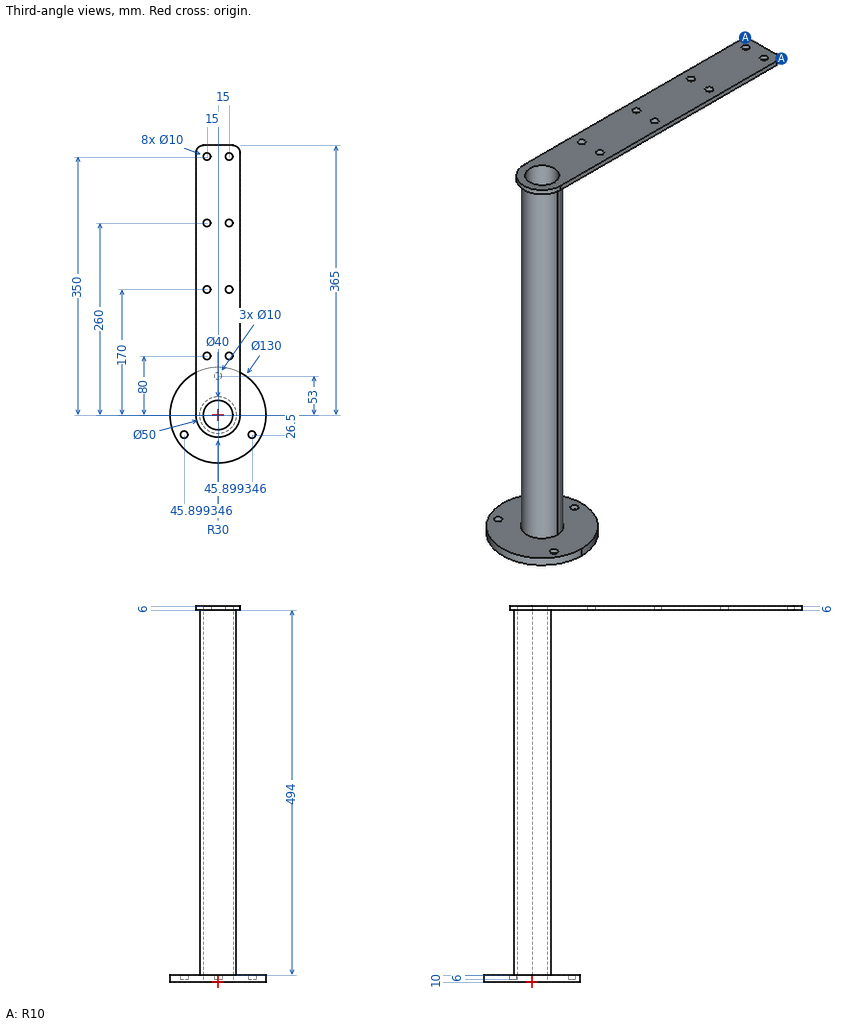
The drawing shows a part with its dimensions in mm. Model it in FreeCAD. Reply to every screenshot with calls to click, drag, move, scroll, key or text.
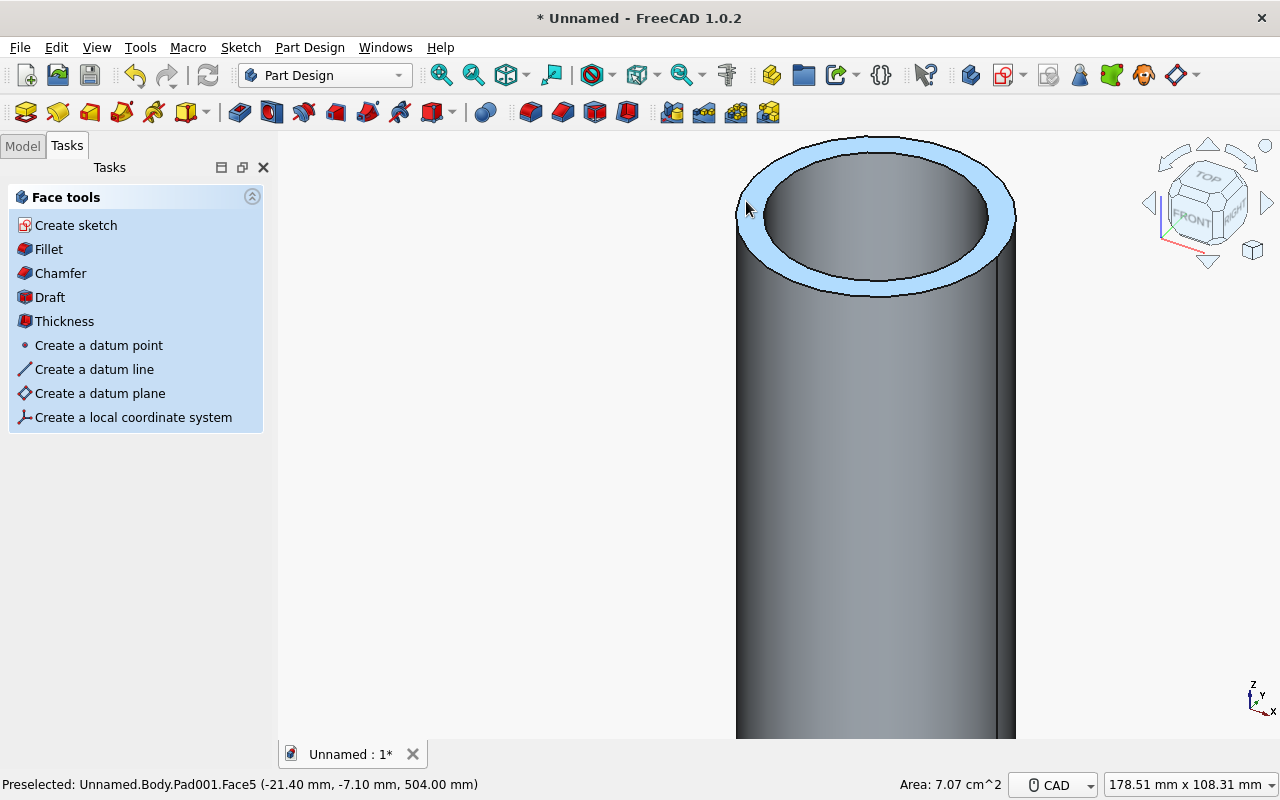
click(1004, 76)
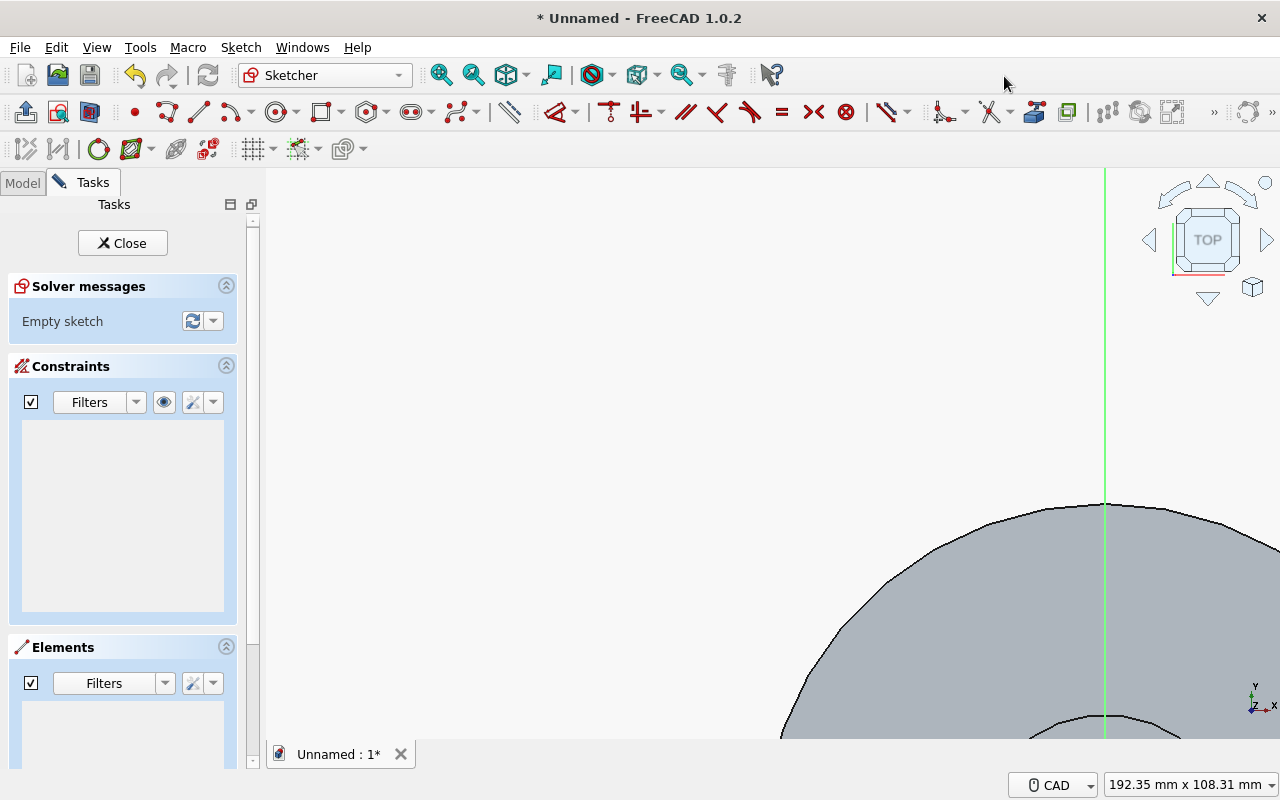
scroll(625, 551, down, 9)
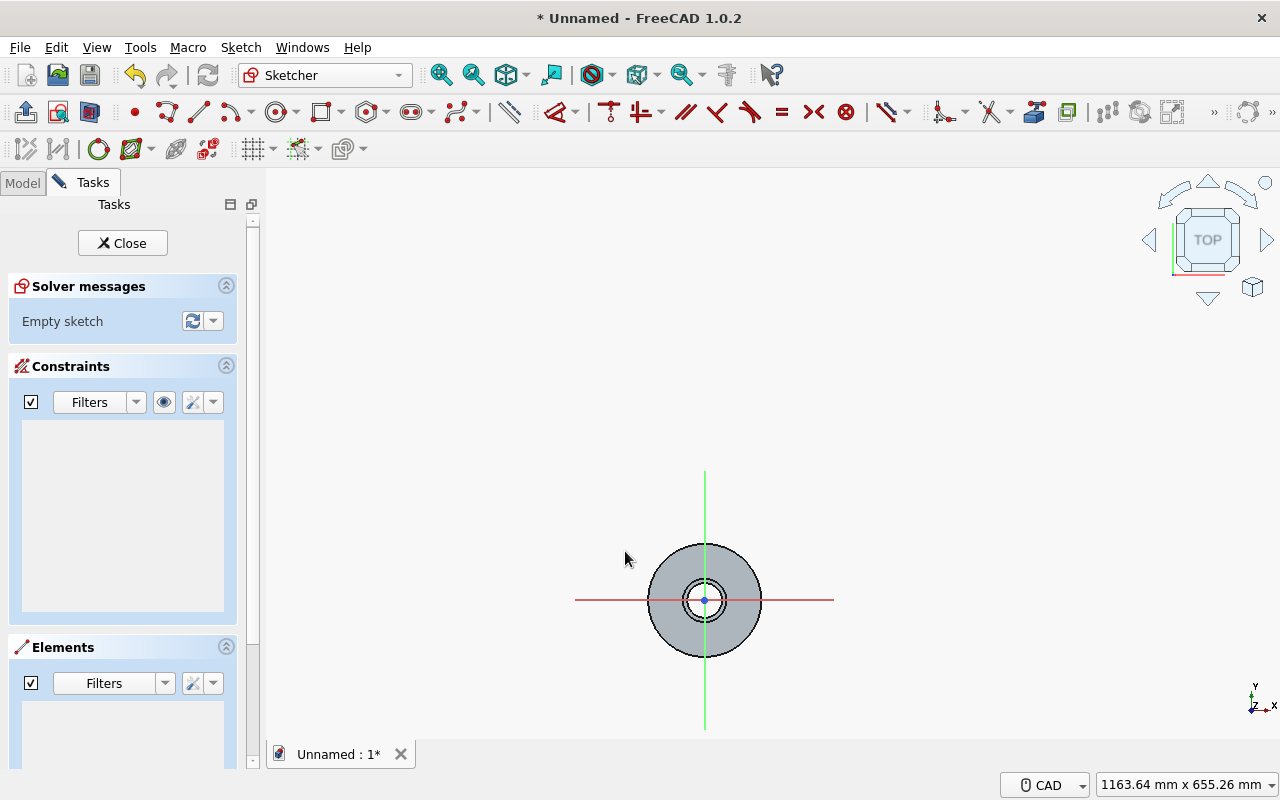
click(168, 112)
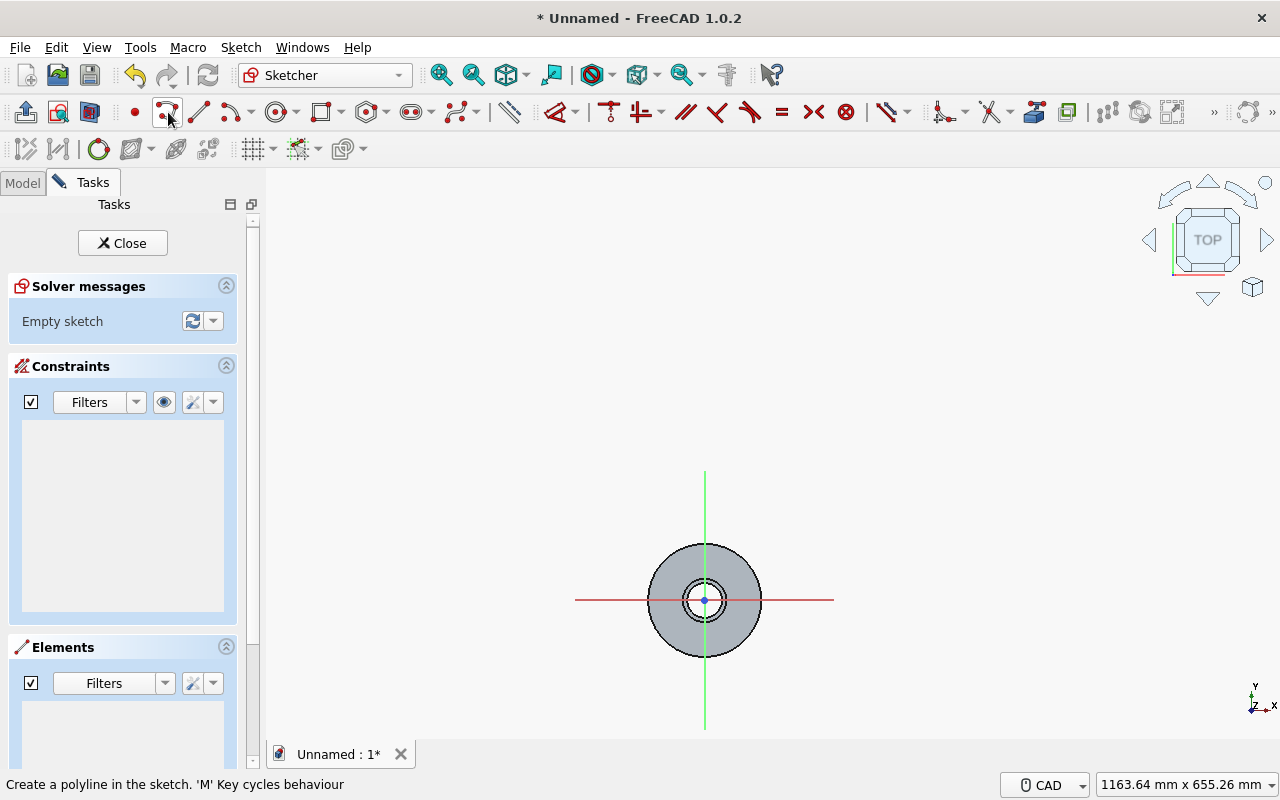
click(731, 600)
click(731, 282)
click(679, 282)
click(679, 600)
right_click(679, 600)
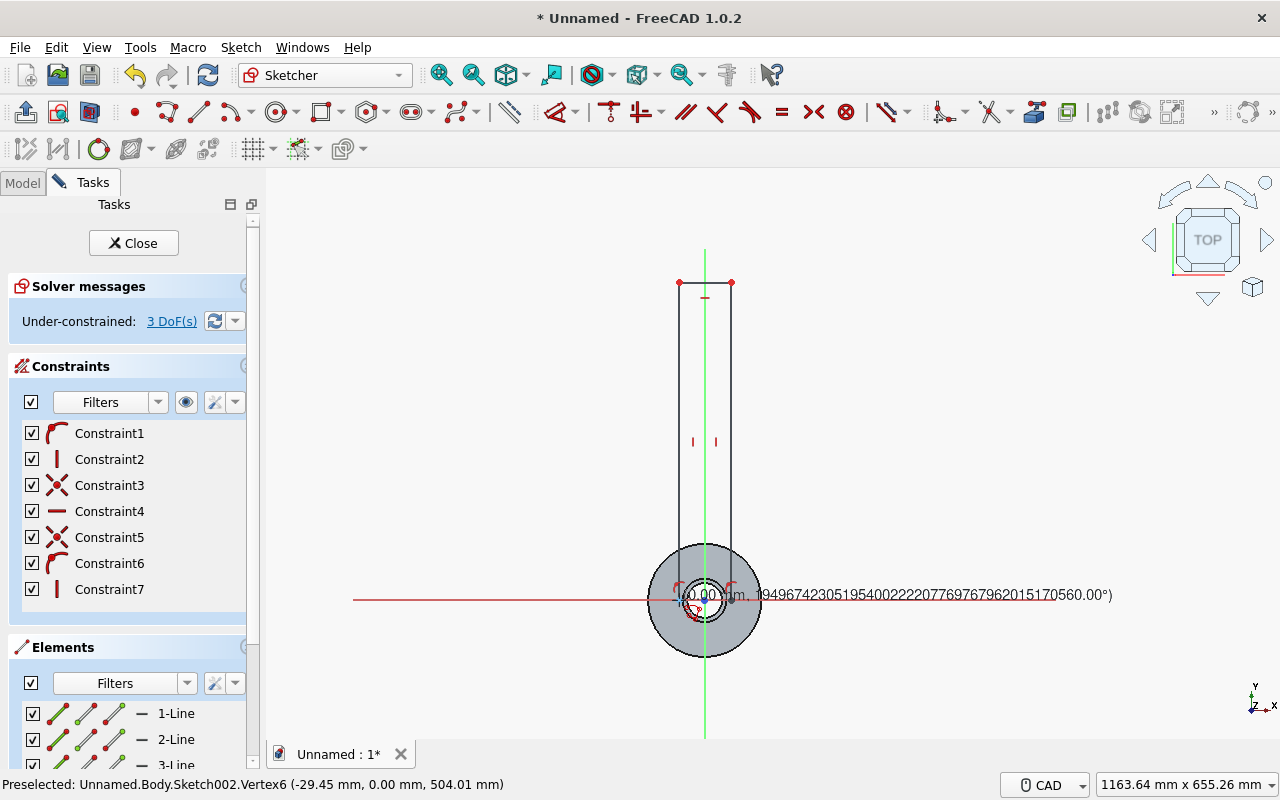
click(254, 112)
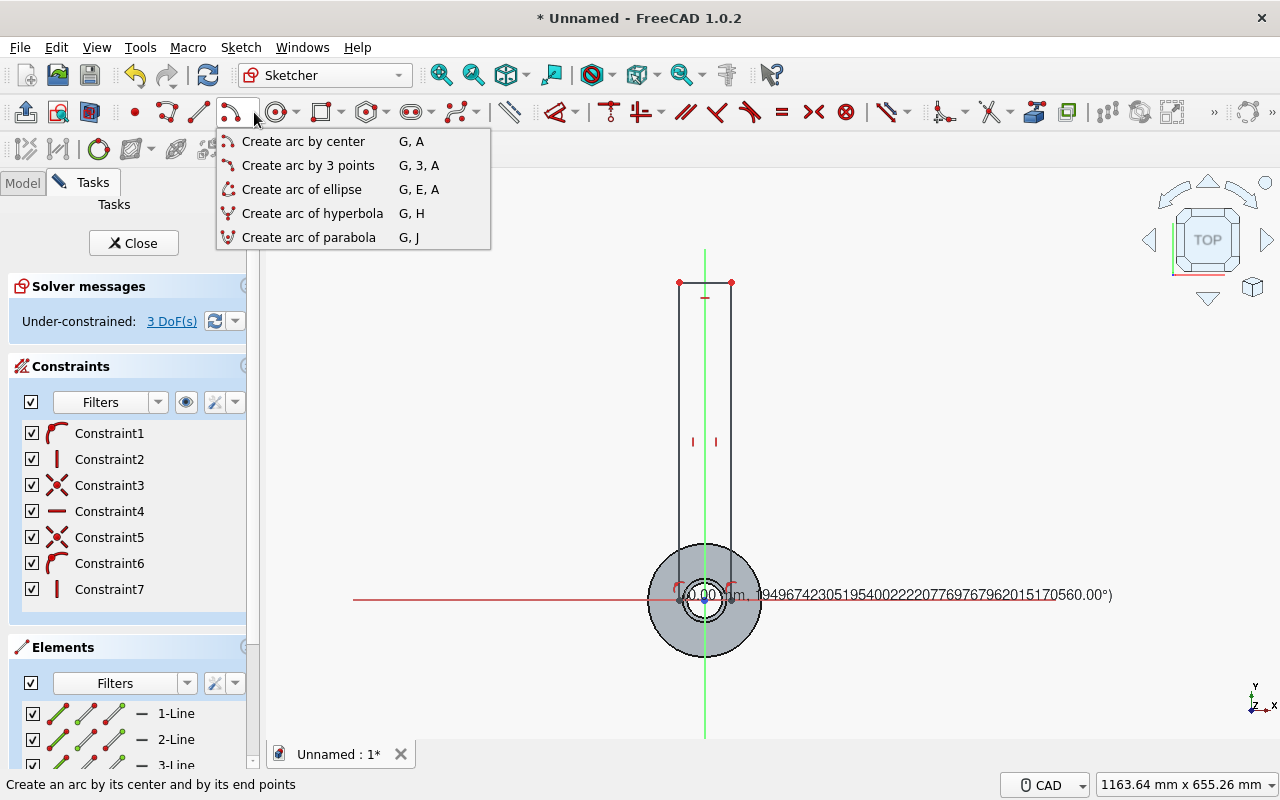
click(354, 165)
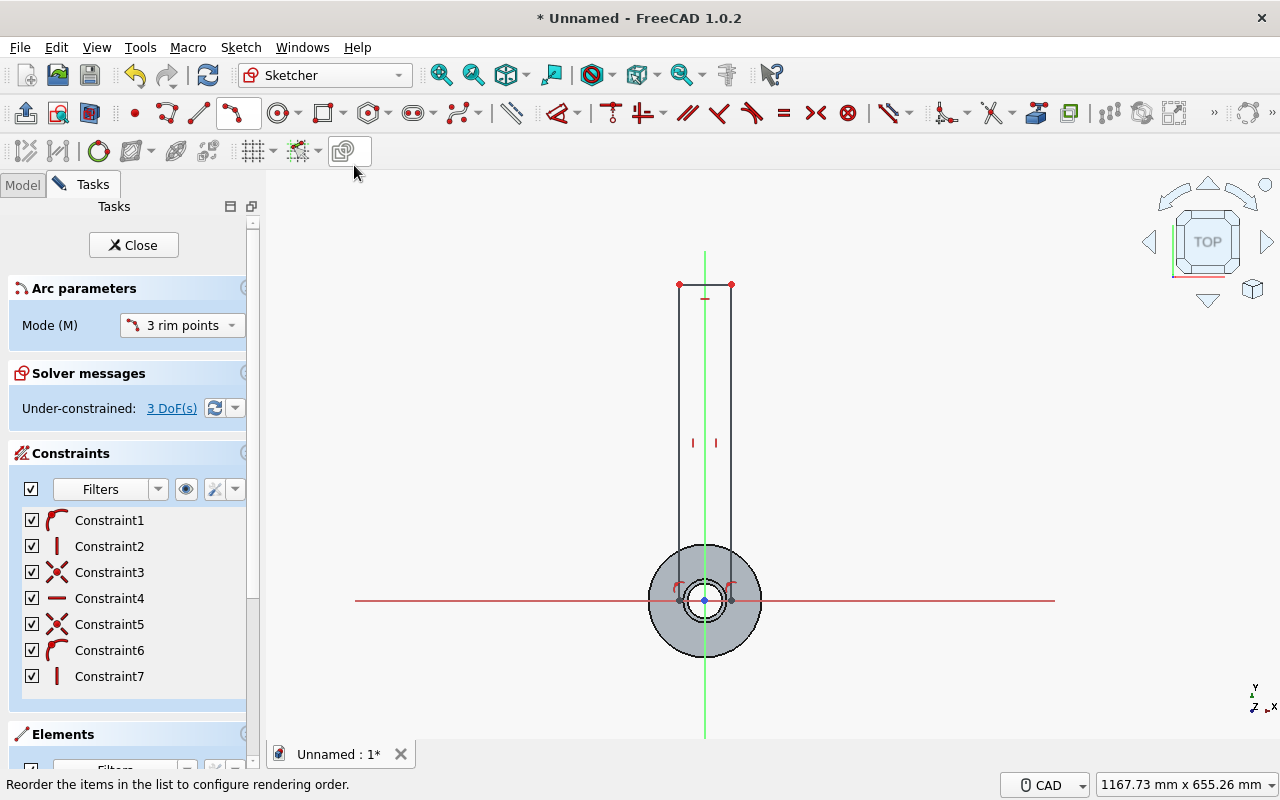
click(679, 601)
click(731, 601)
click(690, 622)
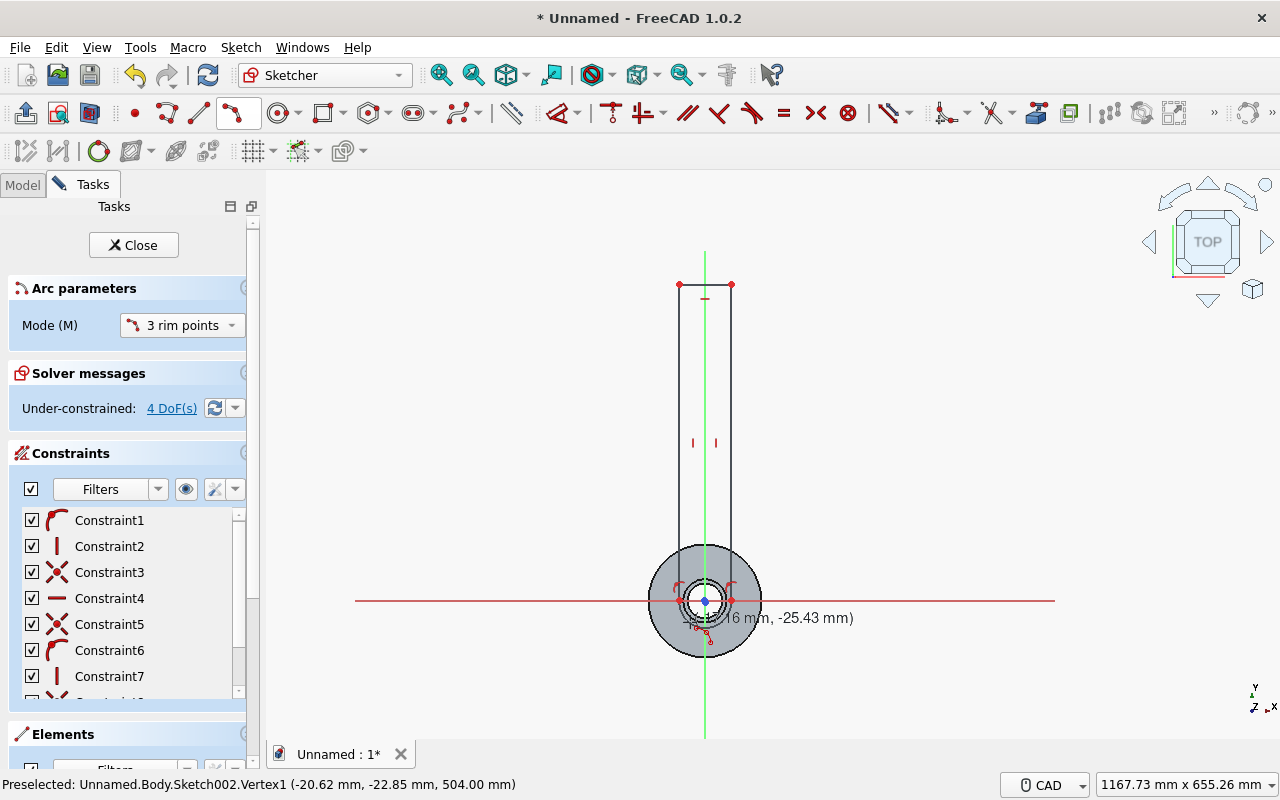
click(278, 114)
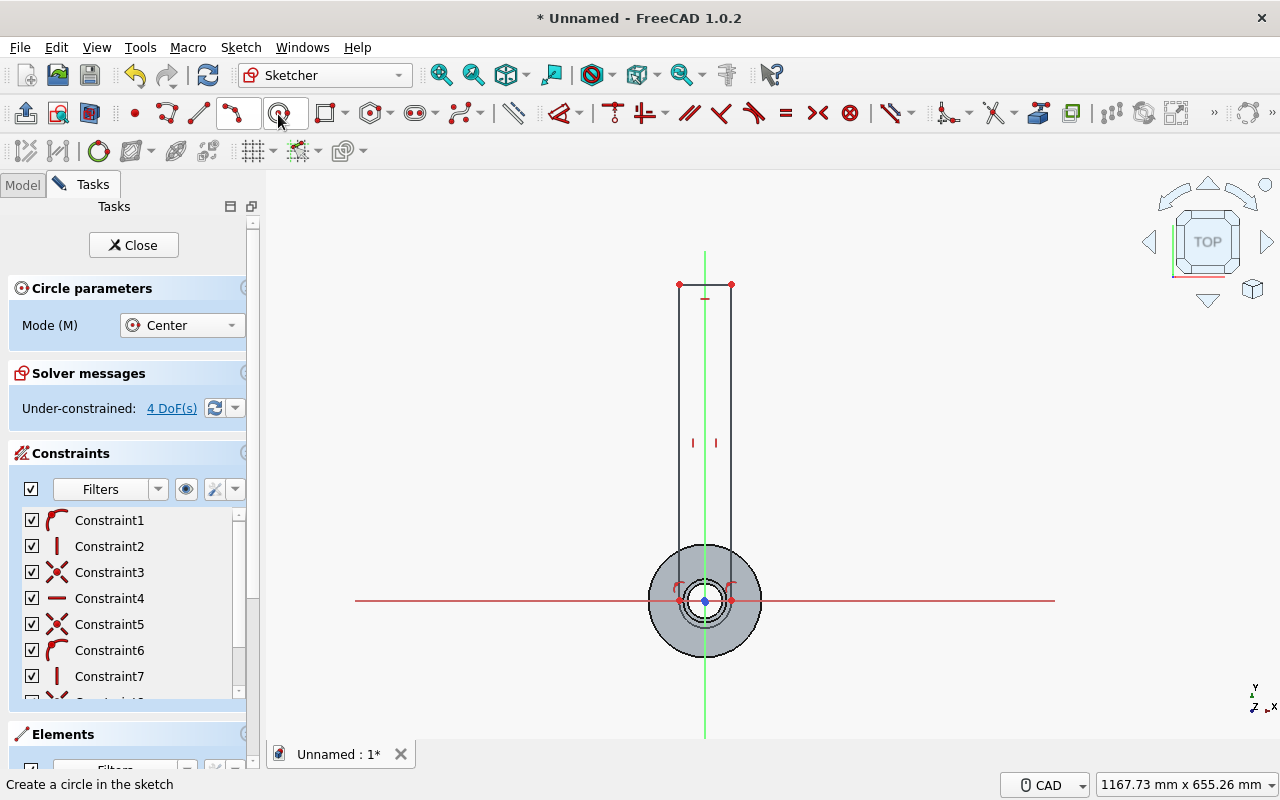
scroll(705, 601, up, 2)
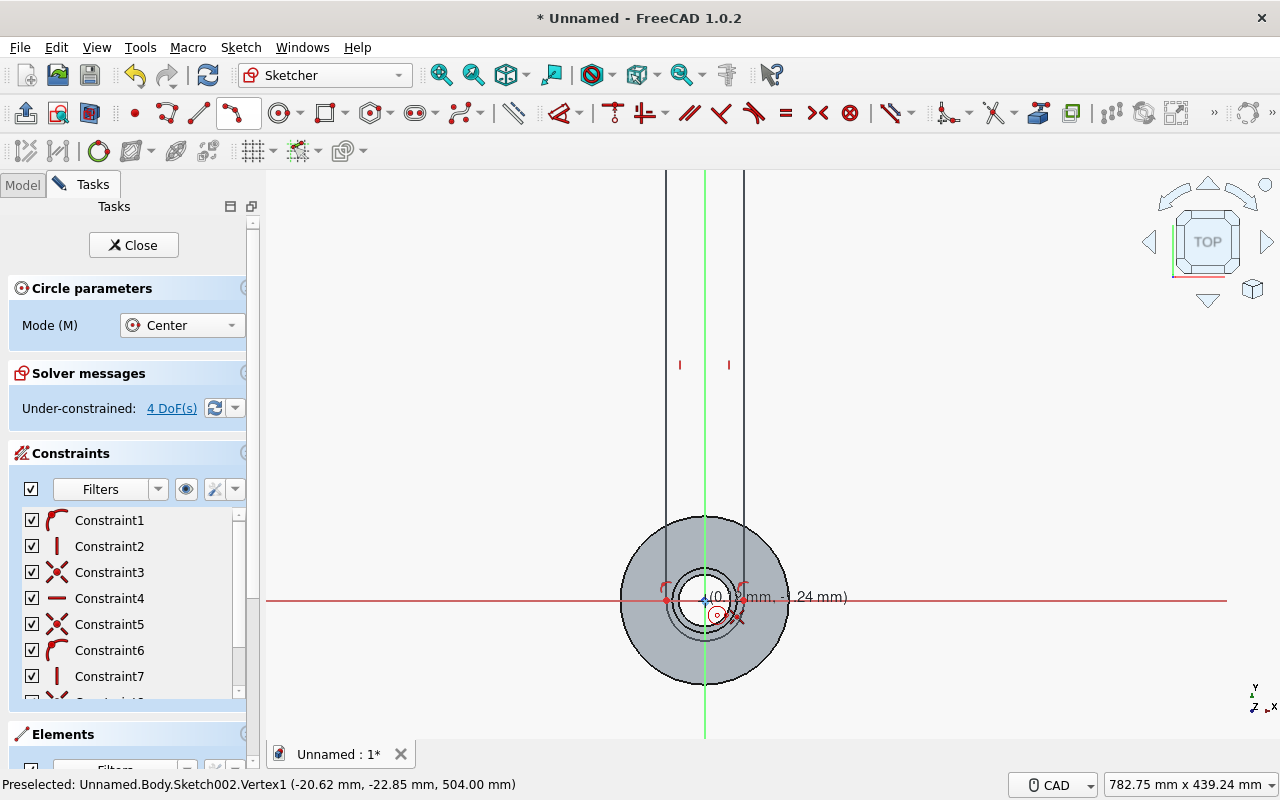
click(705, 601)
move(723, 582)